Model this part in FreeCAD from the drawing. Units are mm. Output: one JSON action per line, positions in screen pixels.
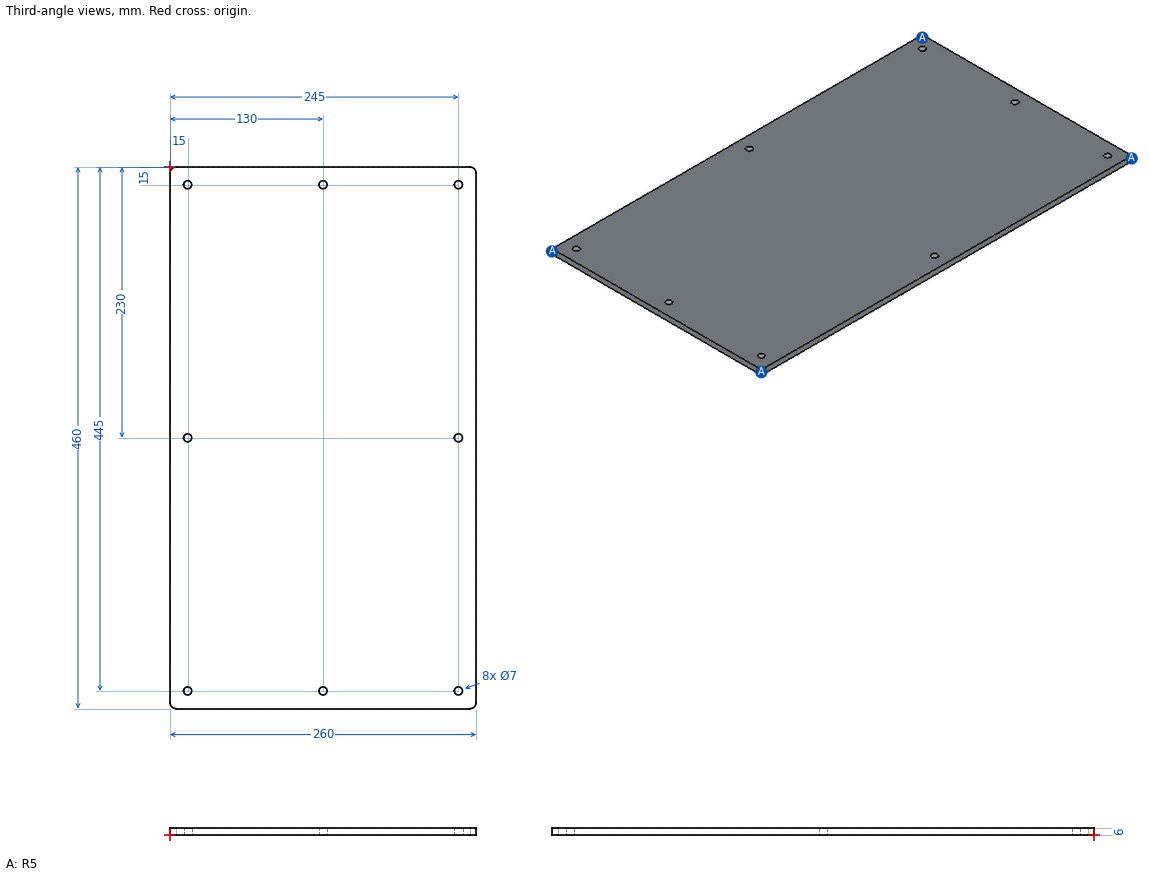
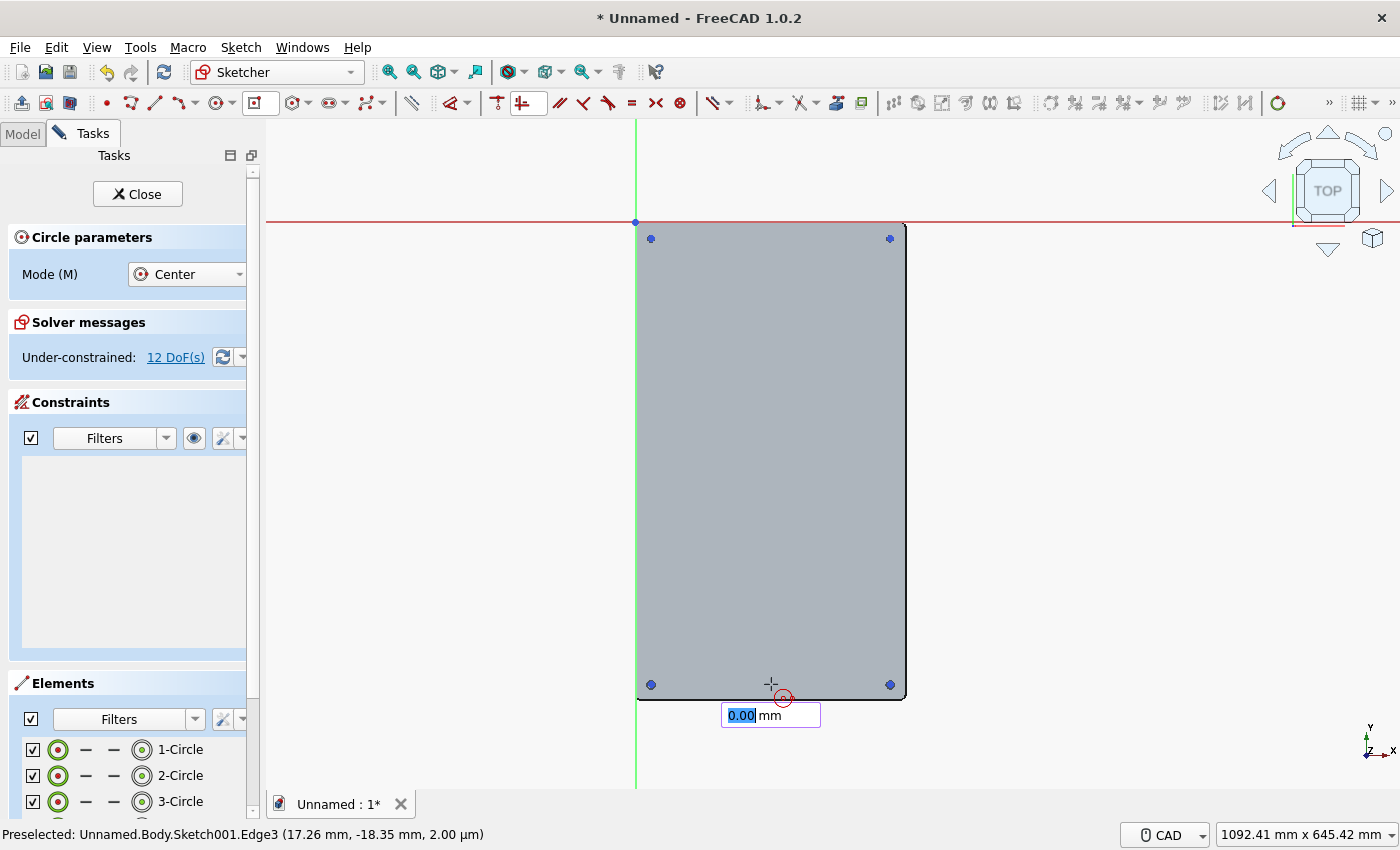
{"action": "scroll", "coordinate": [773, 682], "scroll_direction": "up", "scroll_amount": 8}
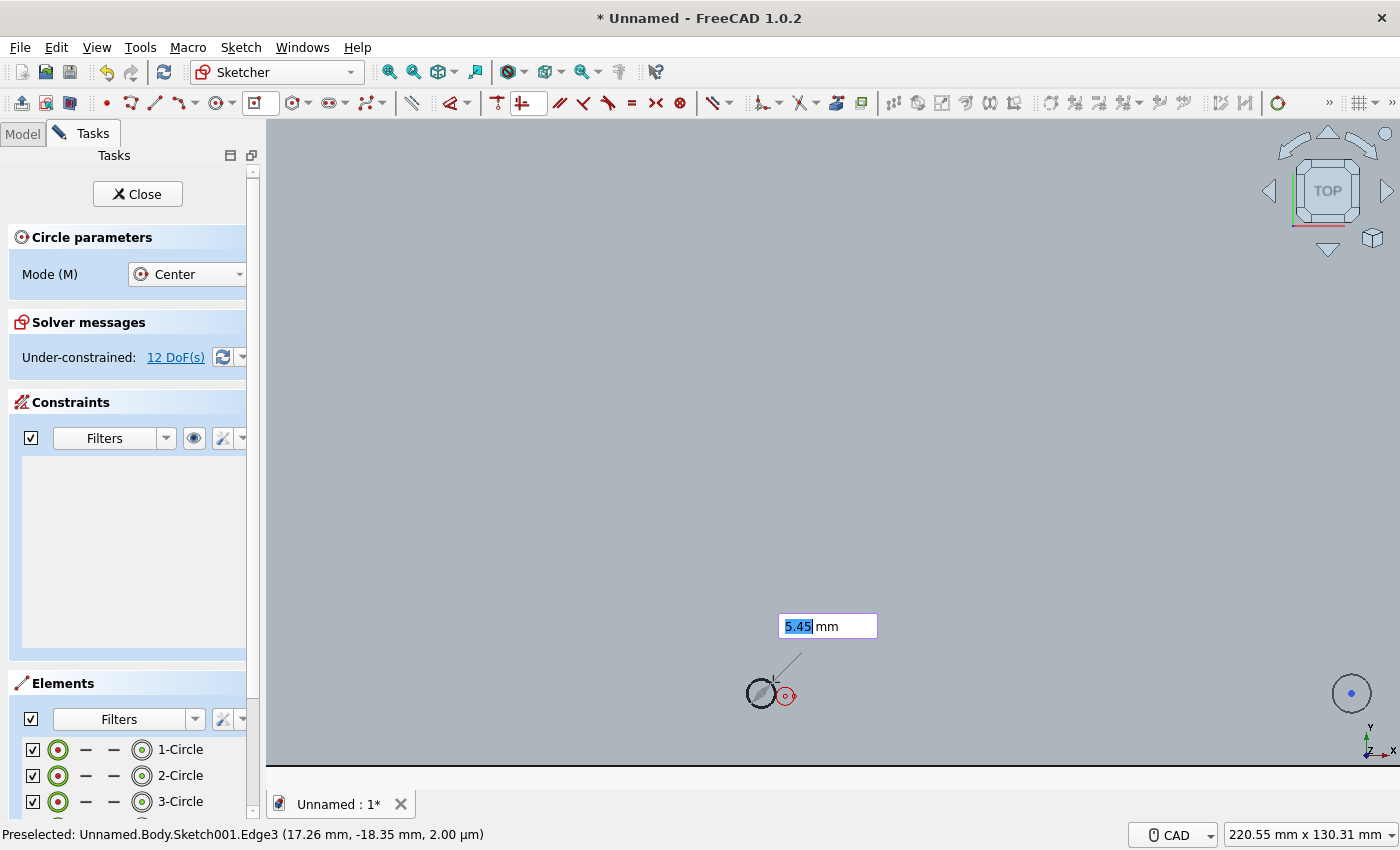
{"action": "left_click", "coordinate": [772, 677]}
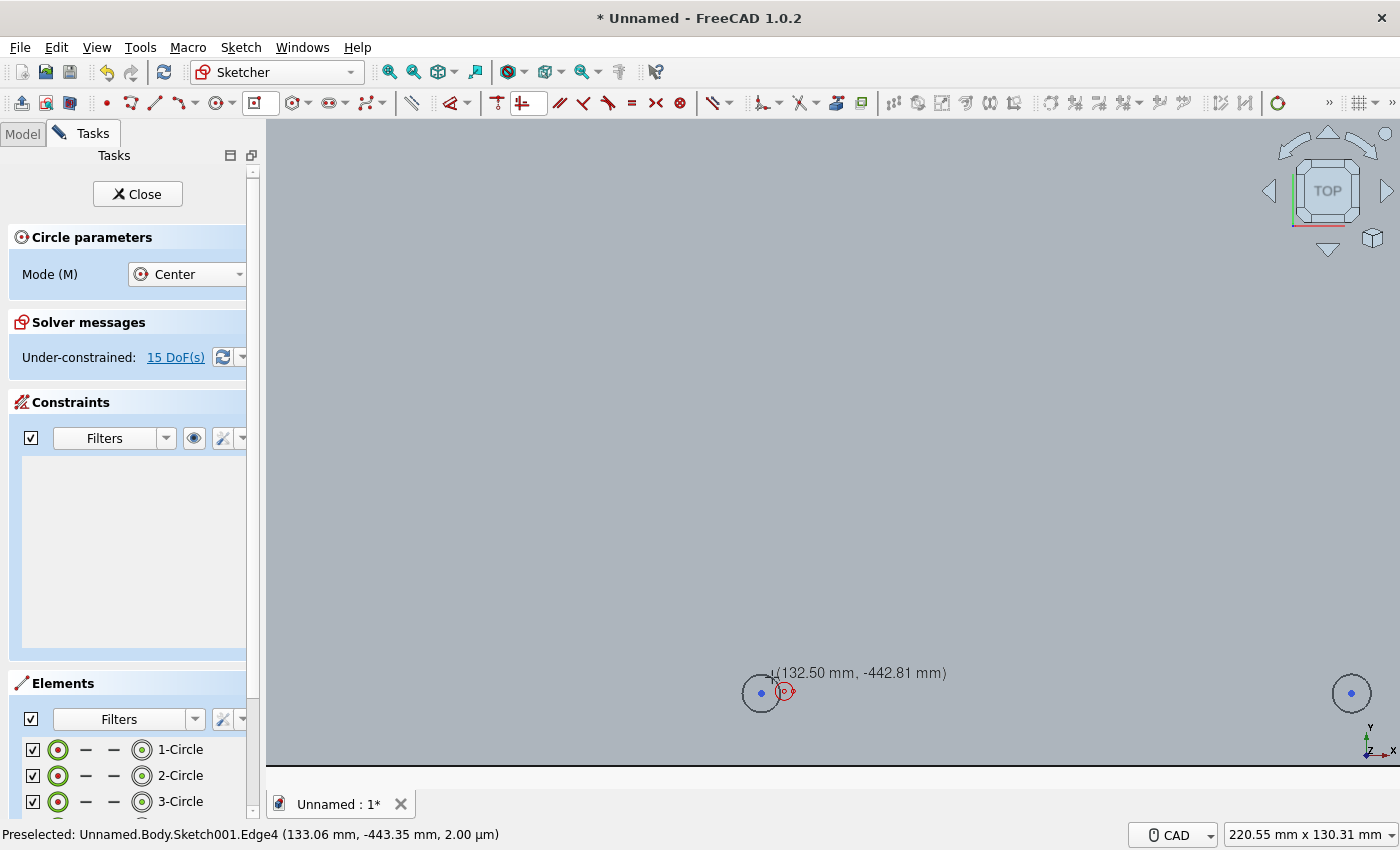
{"action": "scroll", "coordinate": [773, 682], "scroll_direction": "down", "scroll_amount": 8}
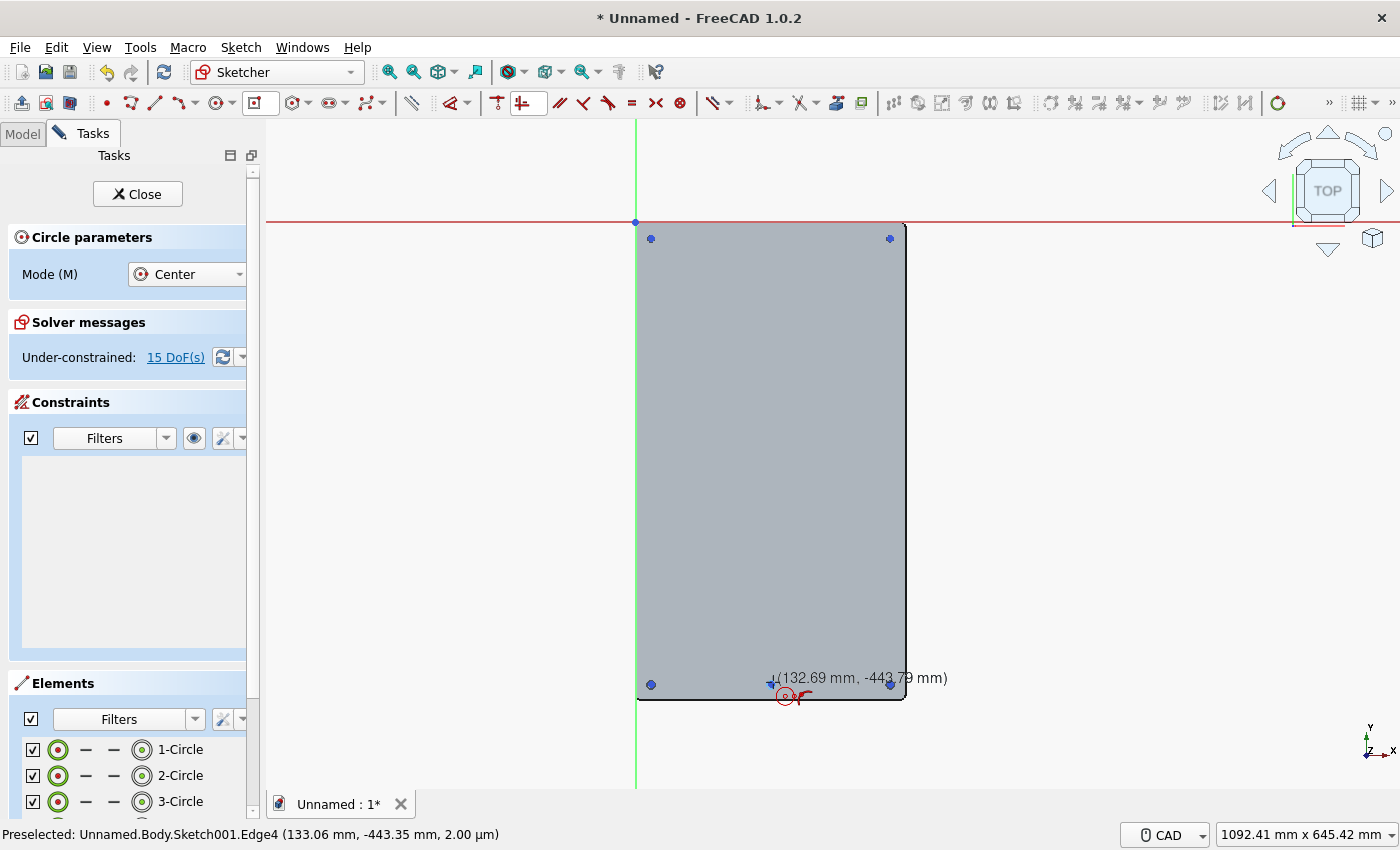
{"action": "scroll", "coordinate": [890, 461], "scroll_direction": "up", "scroll_amount": 10}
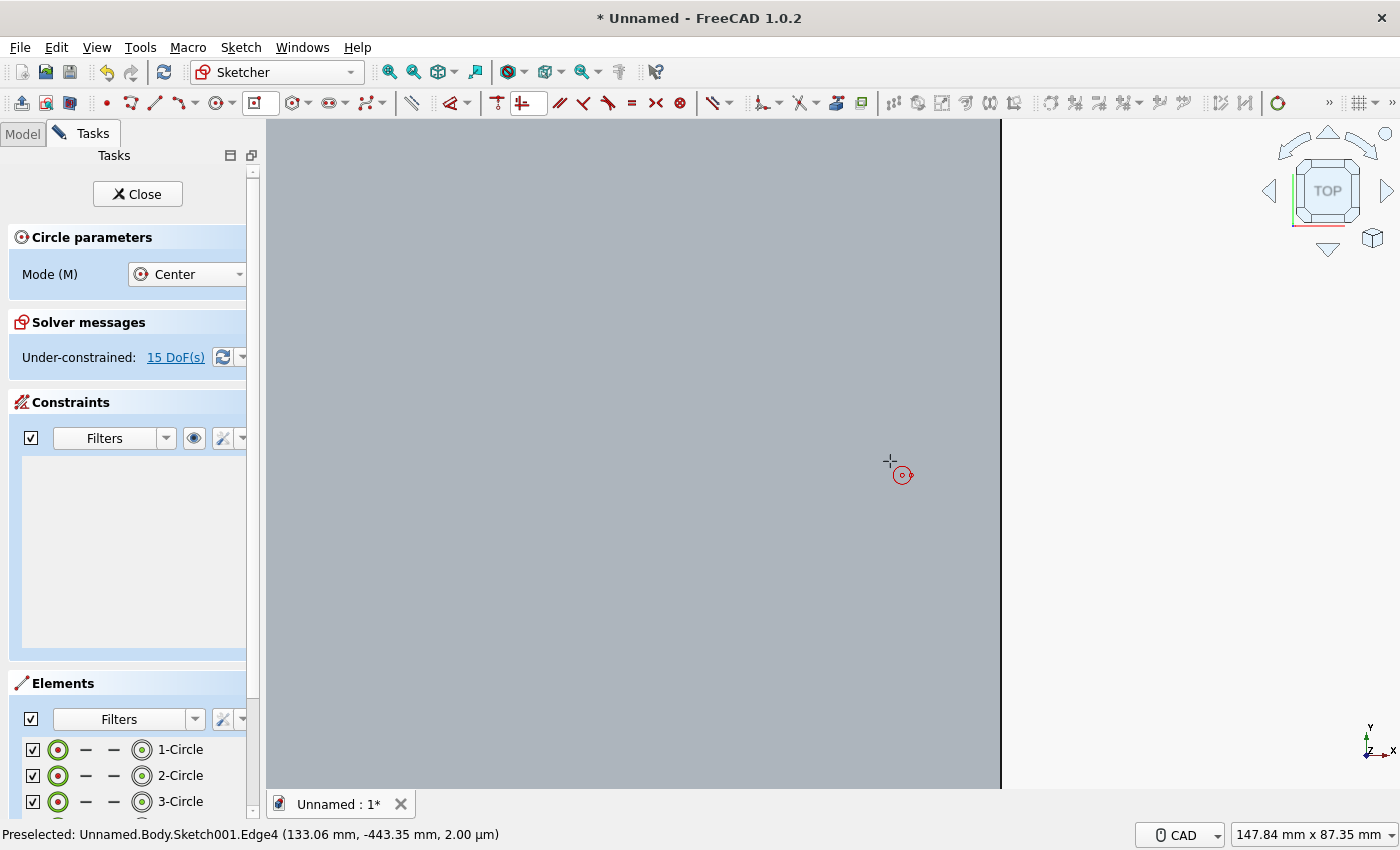
{"action": "scroll", "coordinate": [890, 460], "scroll_direction": "down", "scroll_amount": 10}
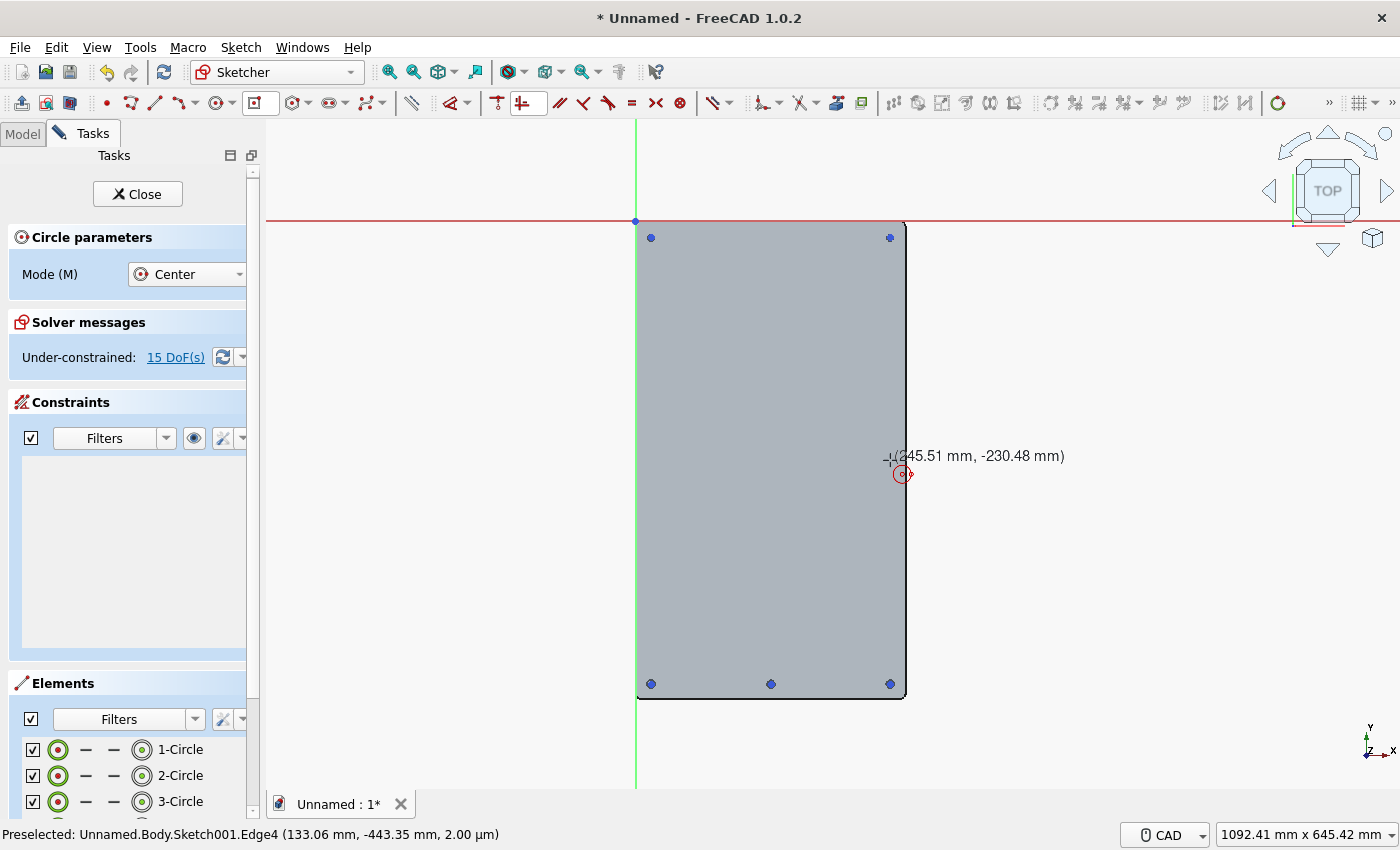
{"action": "left_click", "coordinate": [890, 460]}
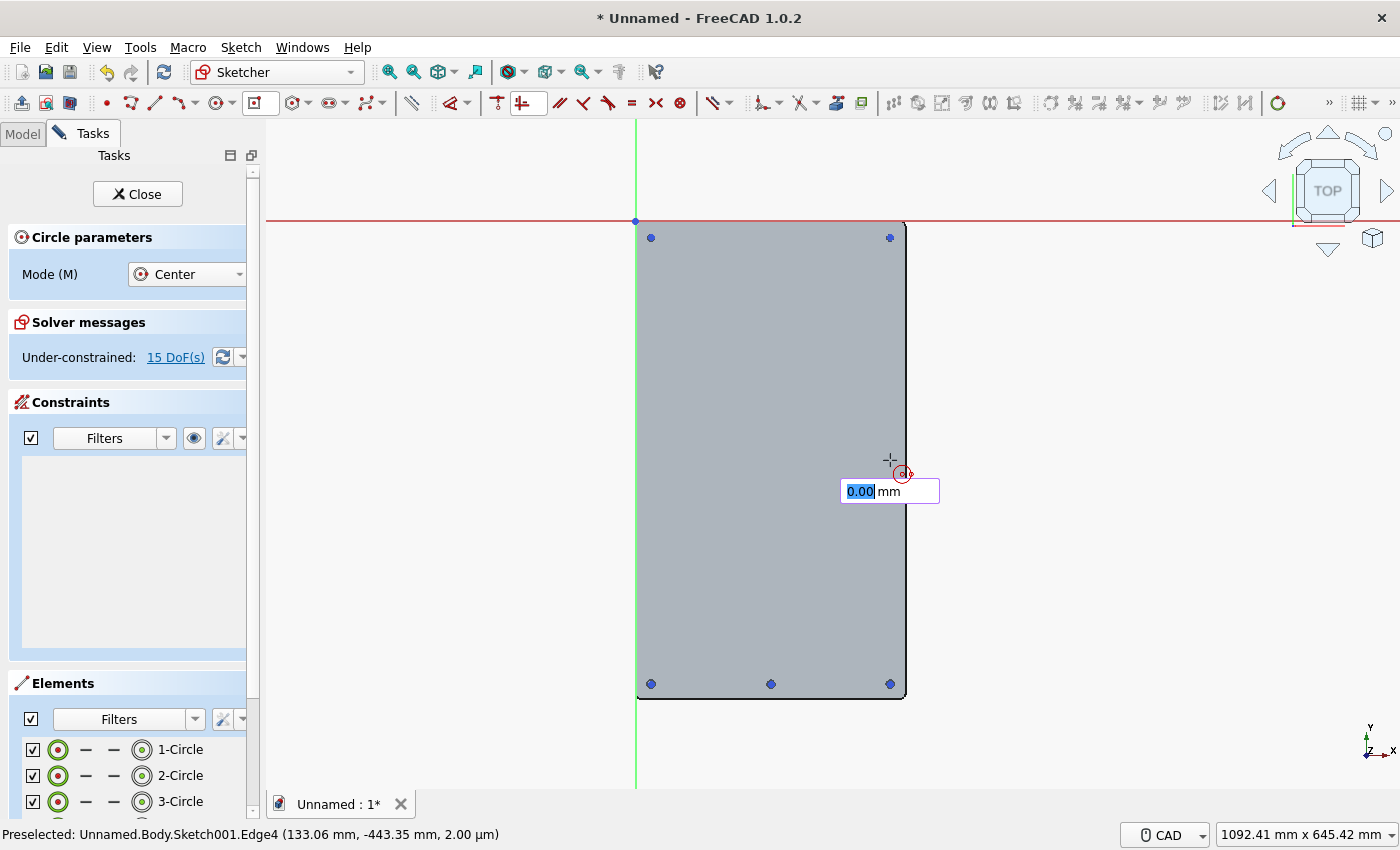
{"action": "scroll", "coordinate": [893, 458], "scroll_direction": "up", "scroll_amount": 8}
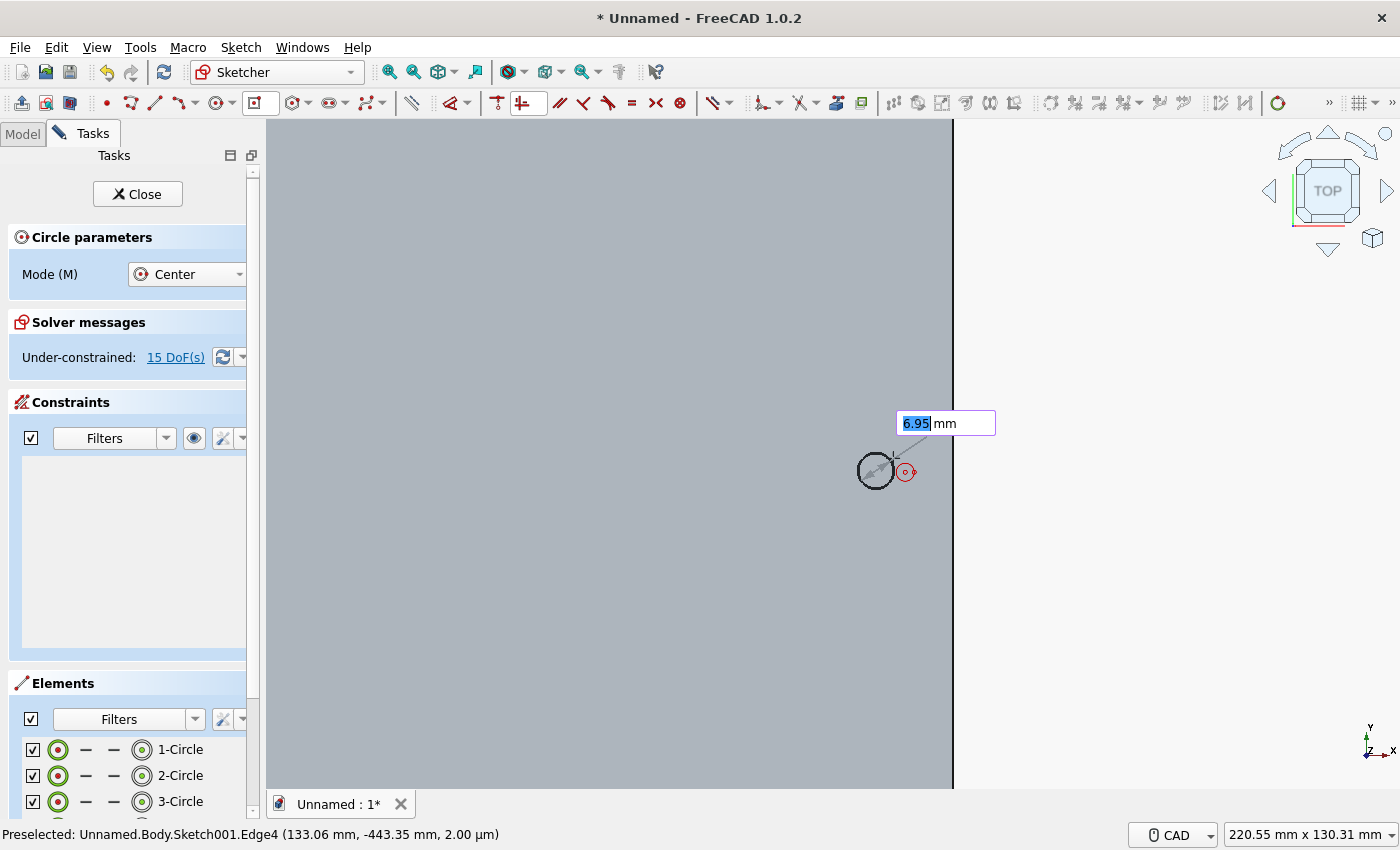
{"action": "left_click", "coordinate": [888, 454]}